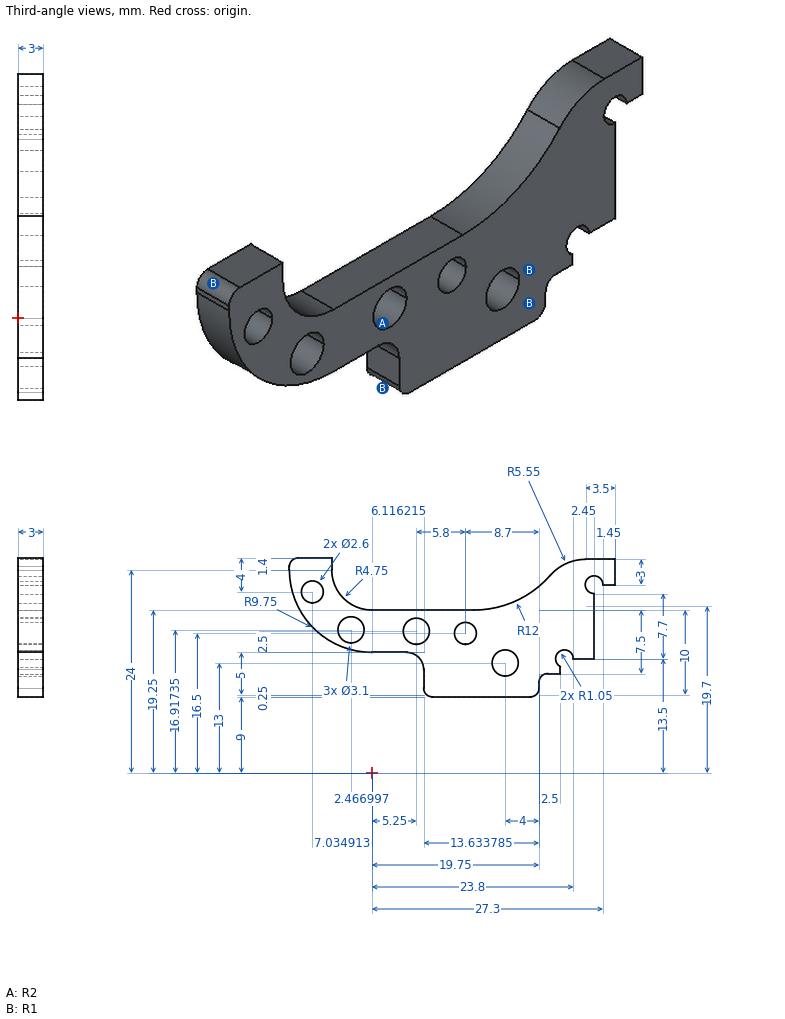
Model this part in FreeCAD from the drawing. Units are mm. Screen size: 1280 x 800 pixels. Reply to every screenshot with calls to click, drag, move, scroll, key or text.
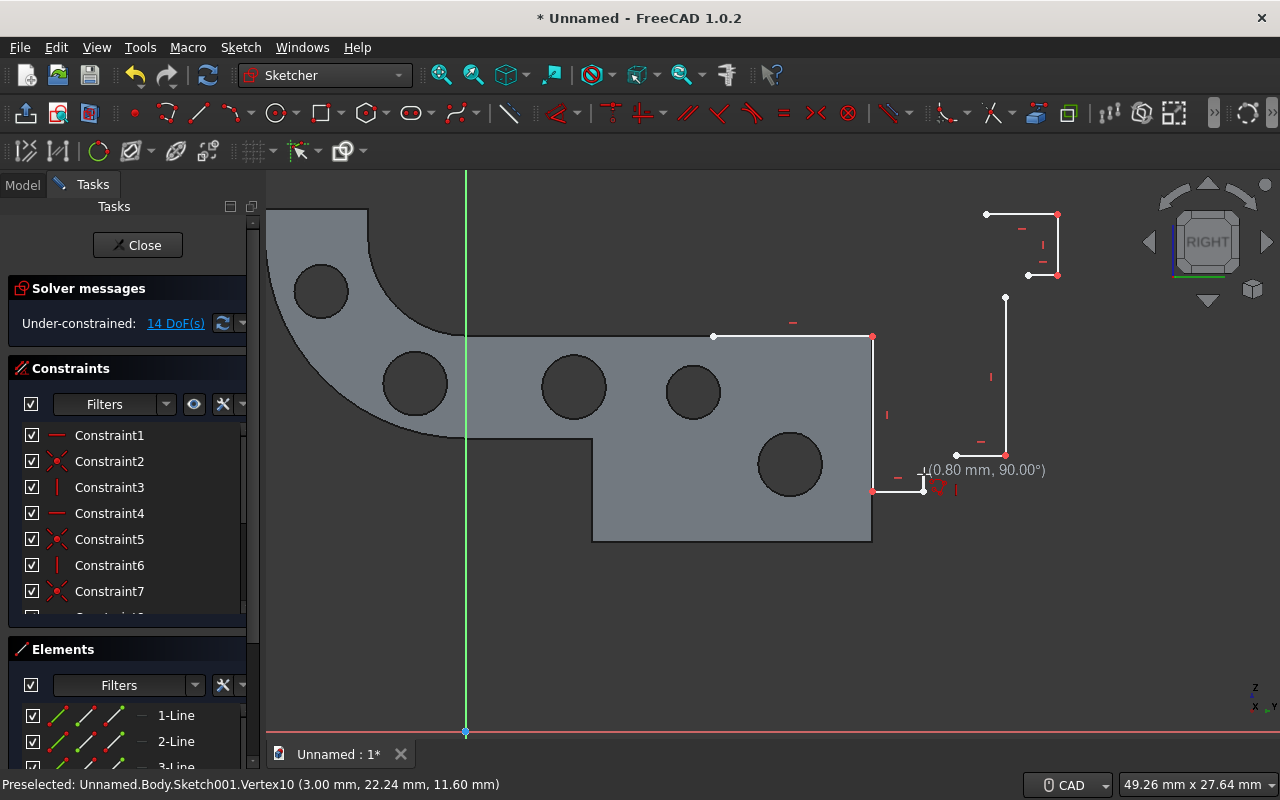
click(924, 473)
right_click(924, 473)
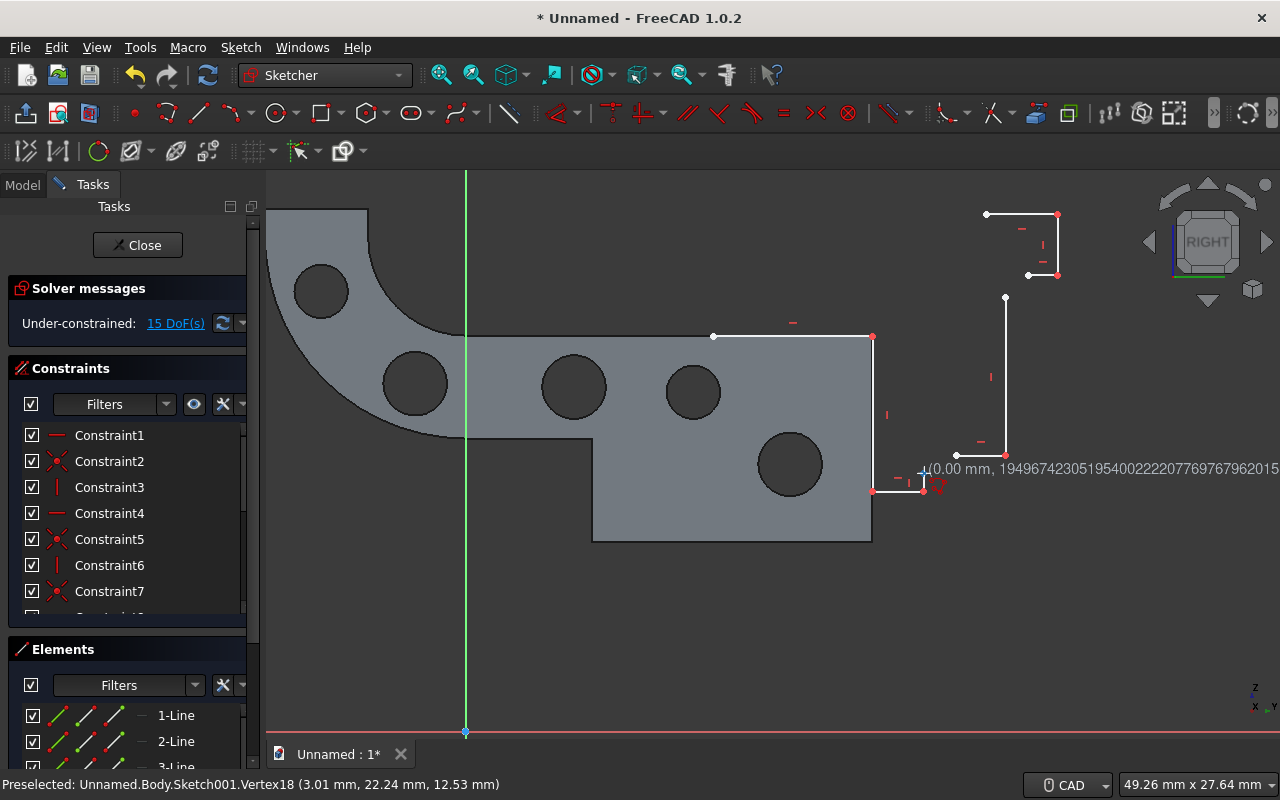
key(g)
key(3)
key(a)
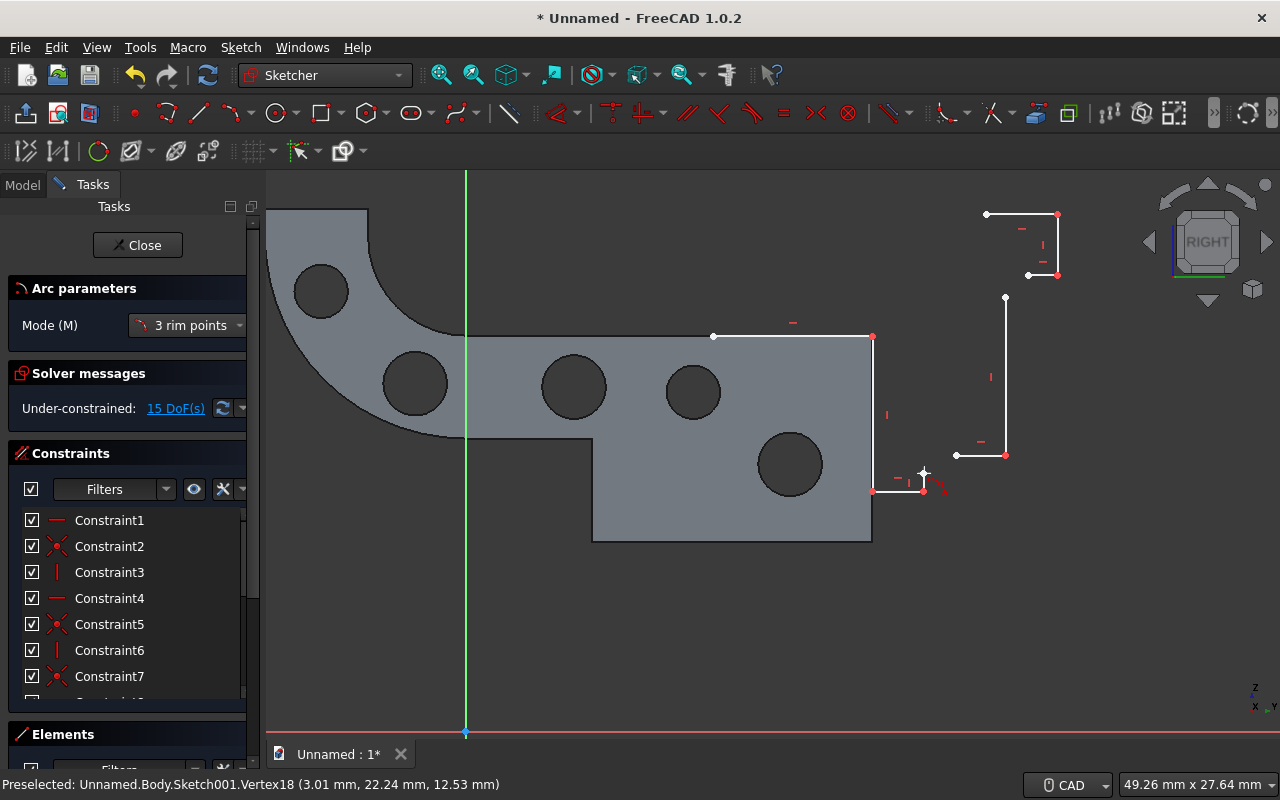
click(1006, 298)
click(1028, 275)
click(991, 259)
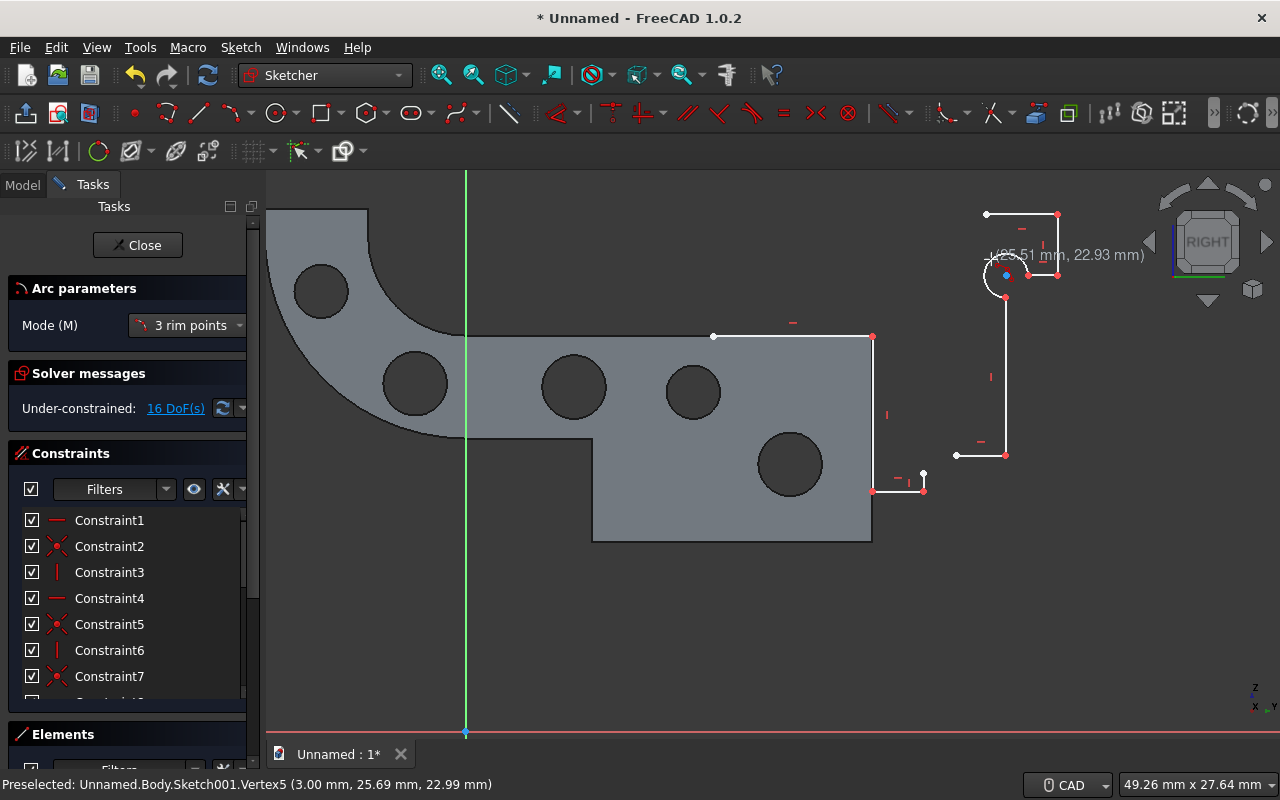
click(986, 214)
click(900, 251)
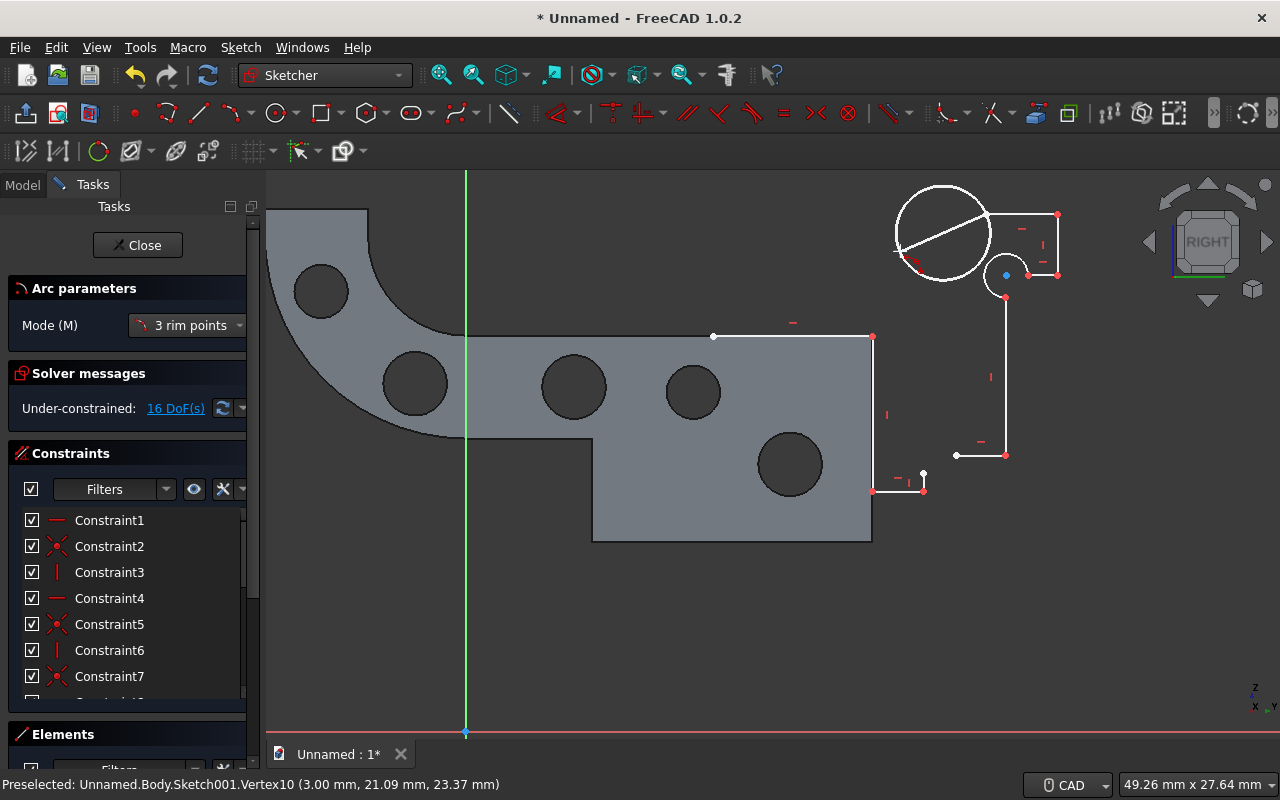
scroll(938, 222, up, 3)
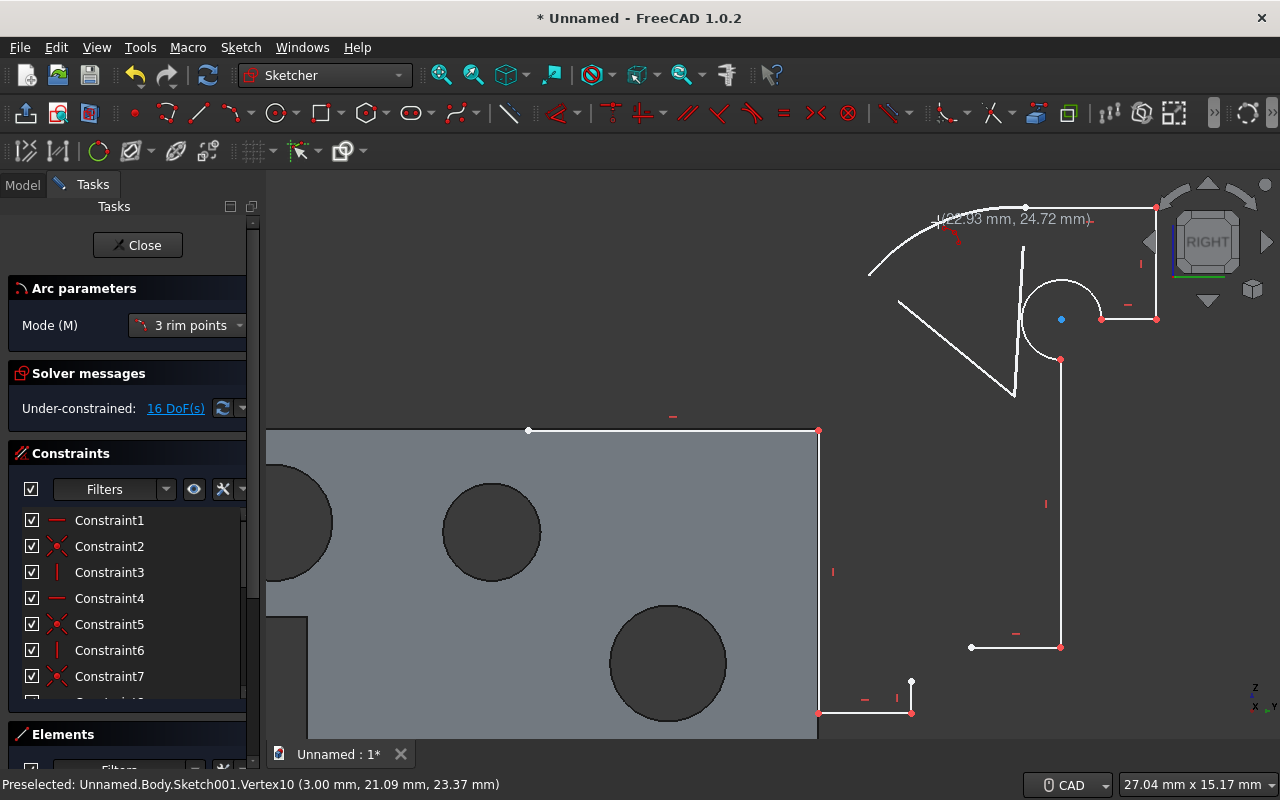
click(938, 223)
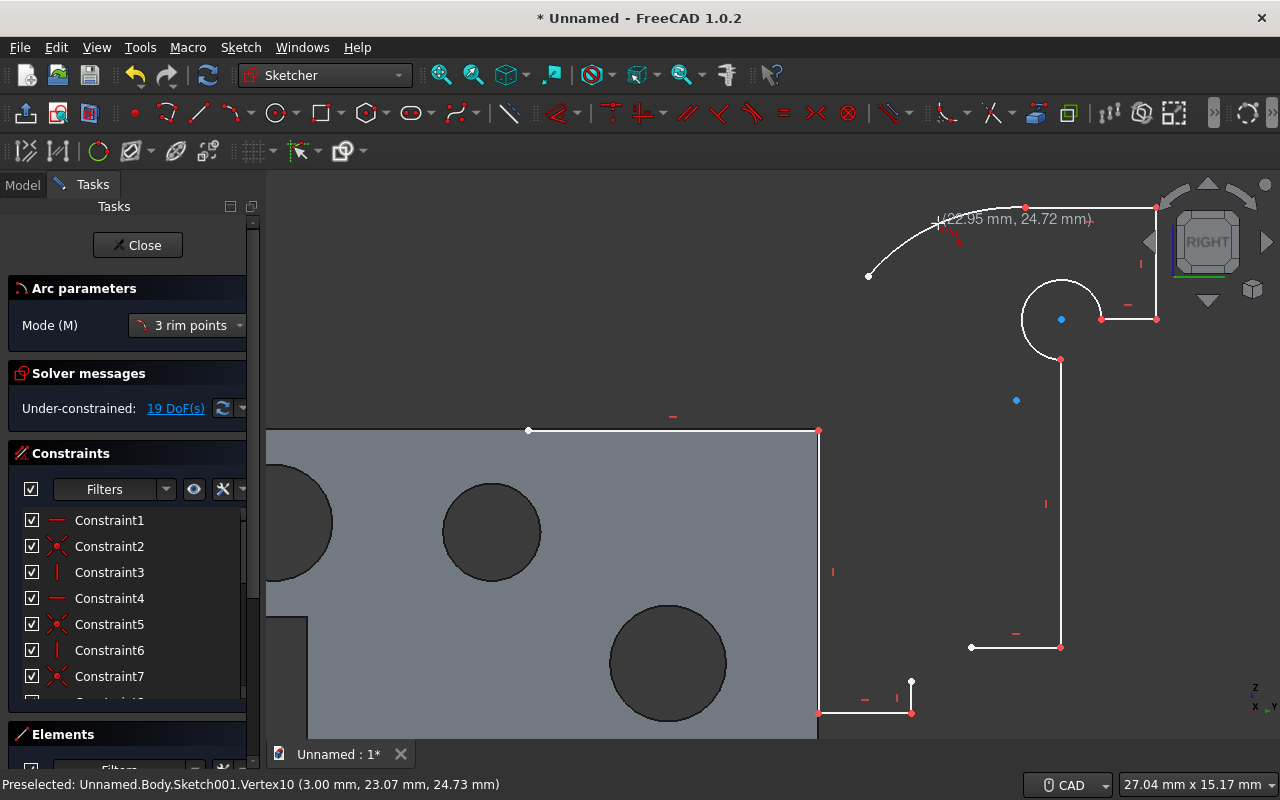
click(868, 277)
click(528, 431)
click(715, 389)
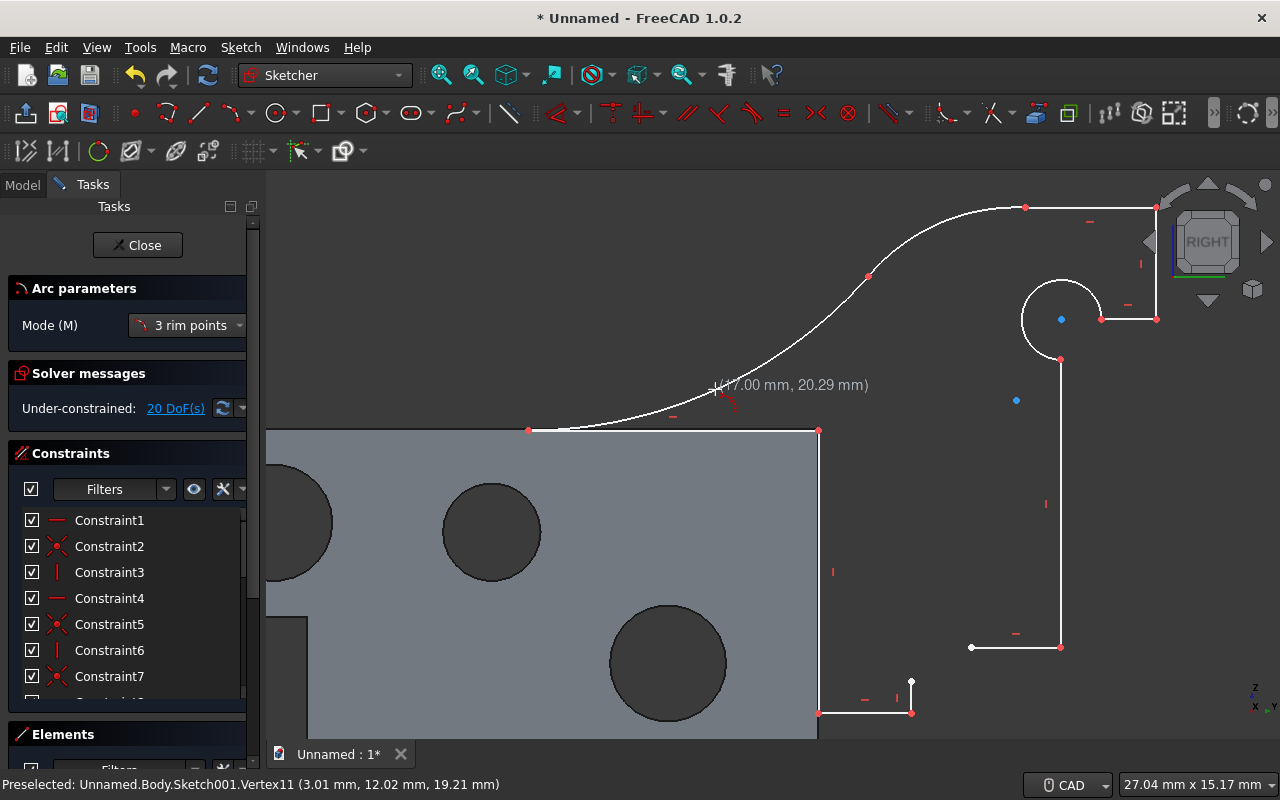
click(911, 681)
click(971, 648)
click(910, 611)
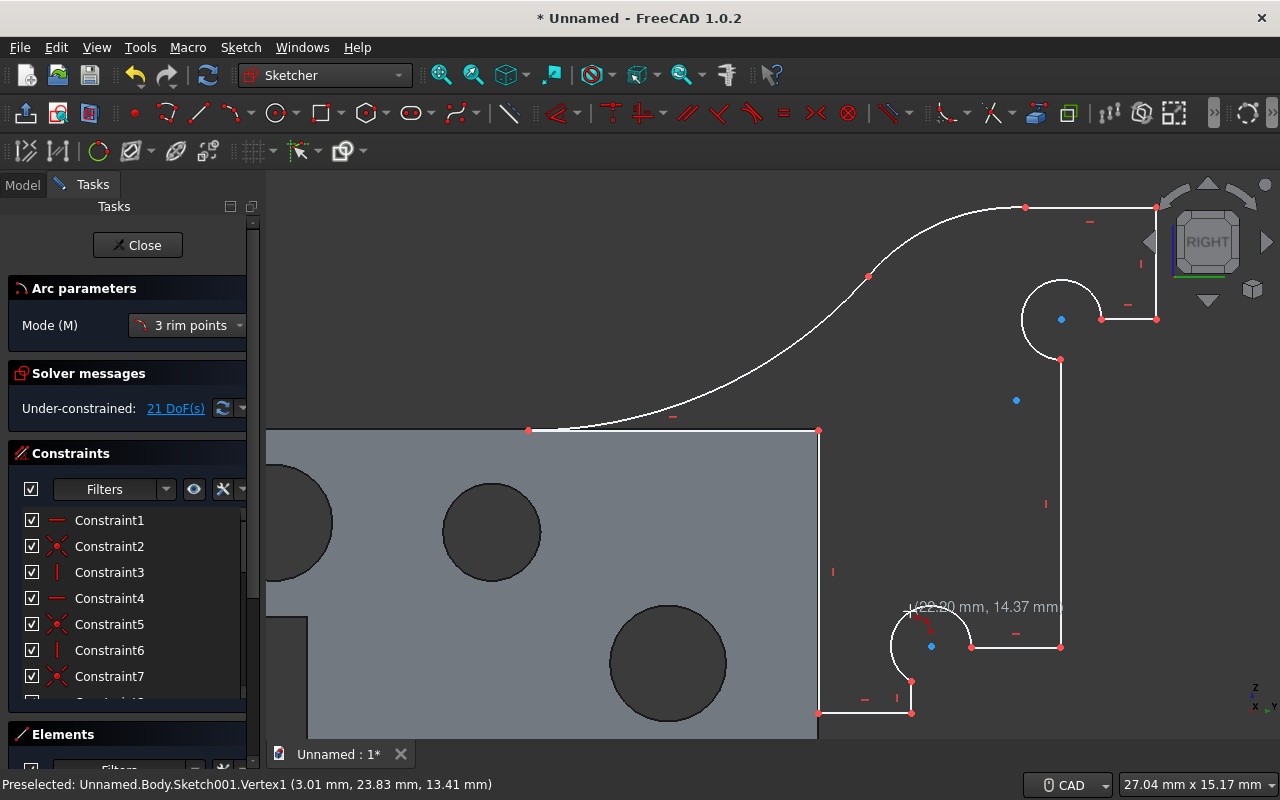
click(322, 114)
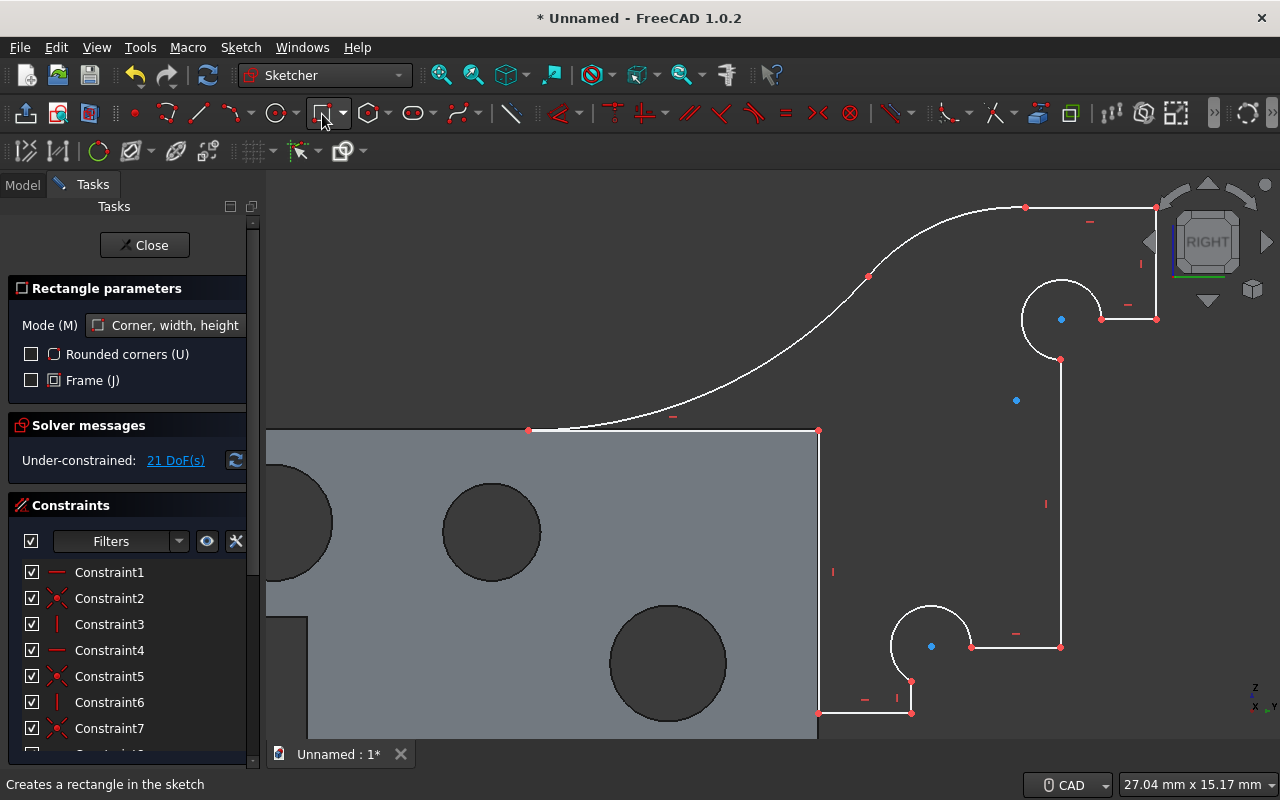
scroll(756, 325, down, 5)